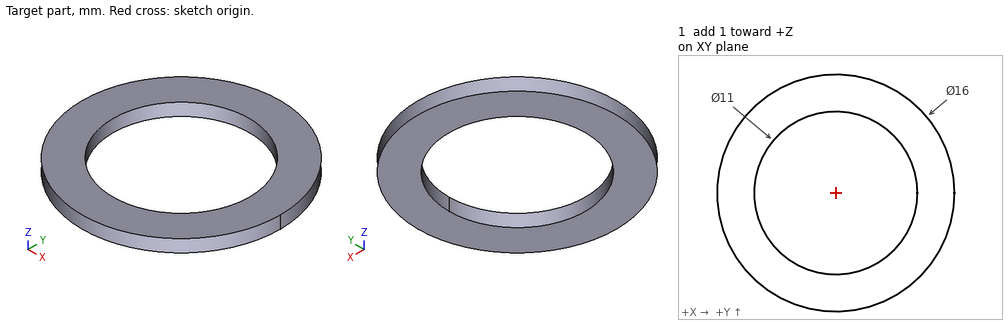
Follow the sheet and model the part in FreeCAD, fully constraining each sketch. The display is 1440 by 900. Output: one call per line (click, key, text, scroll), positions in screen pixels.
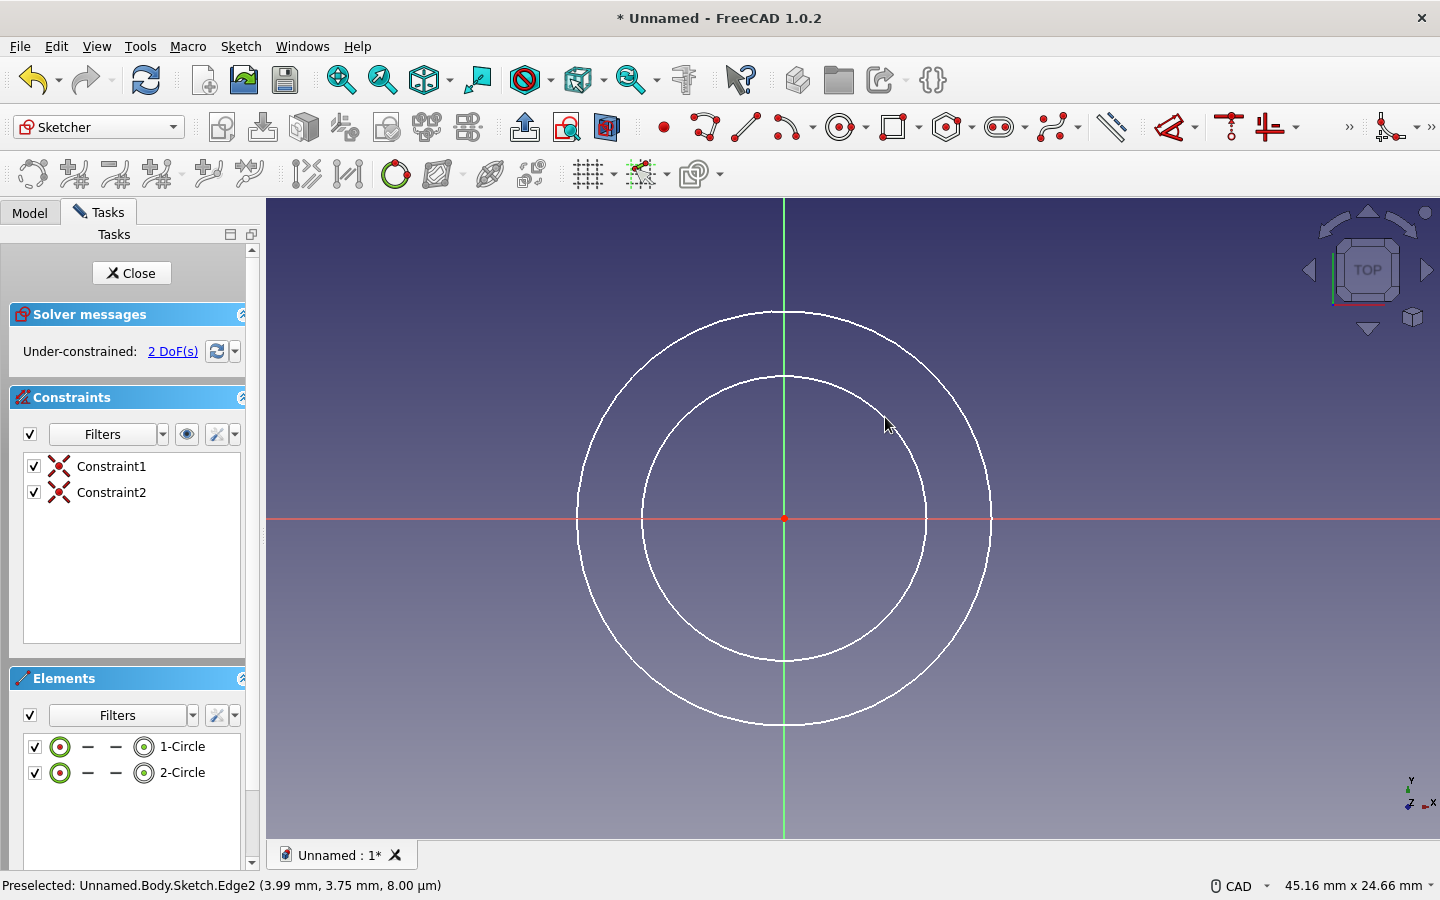
click(930, 371)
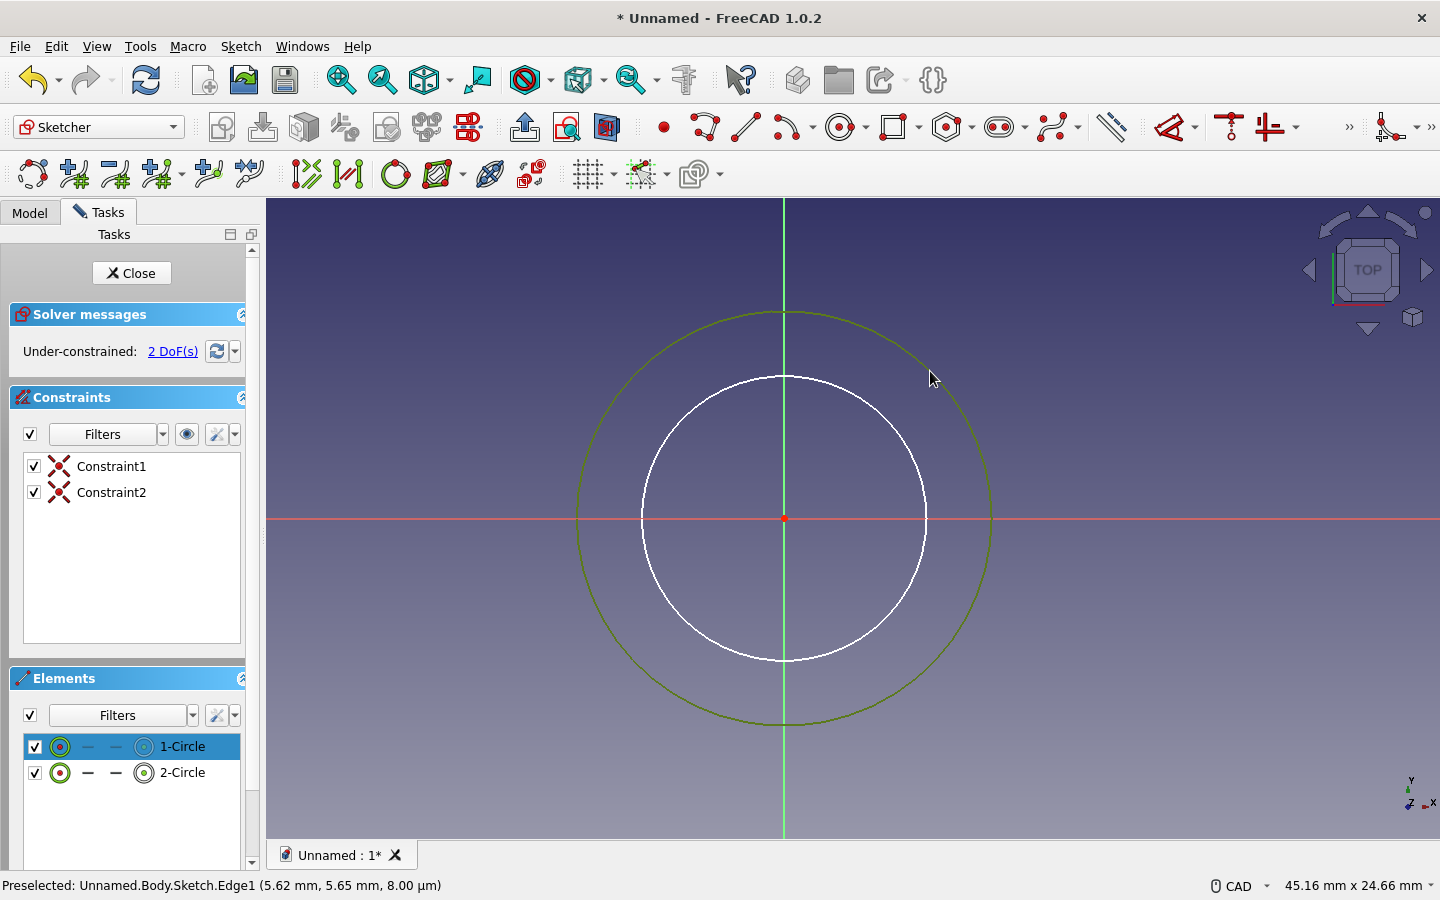
click(1194, 128)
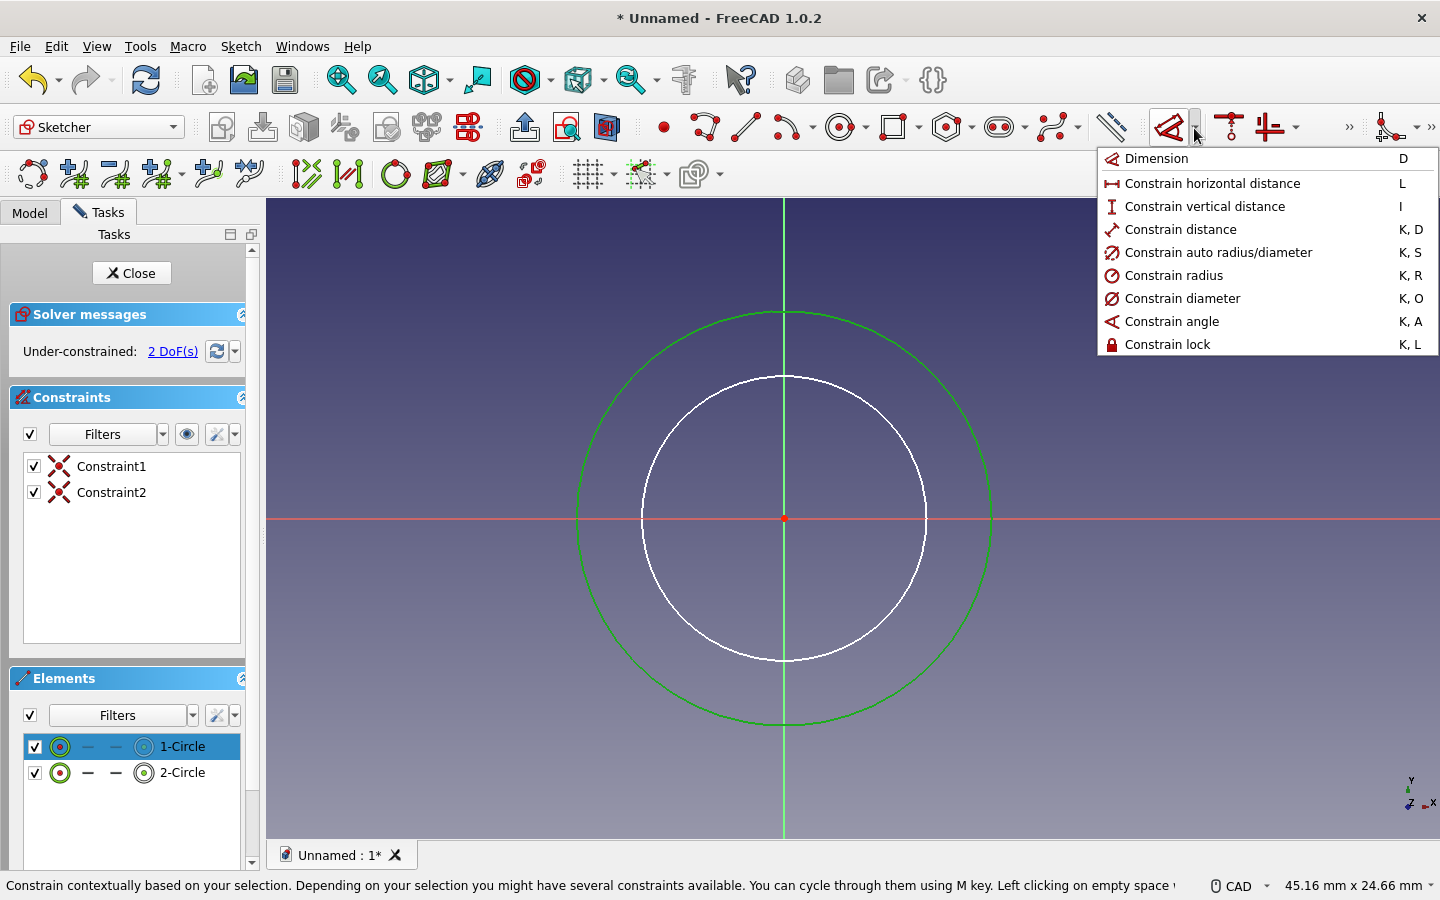
click(1268, 298)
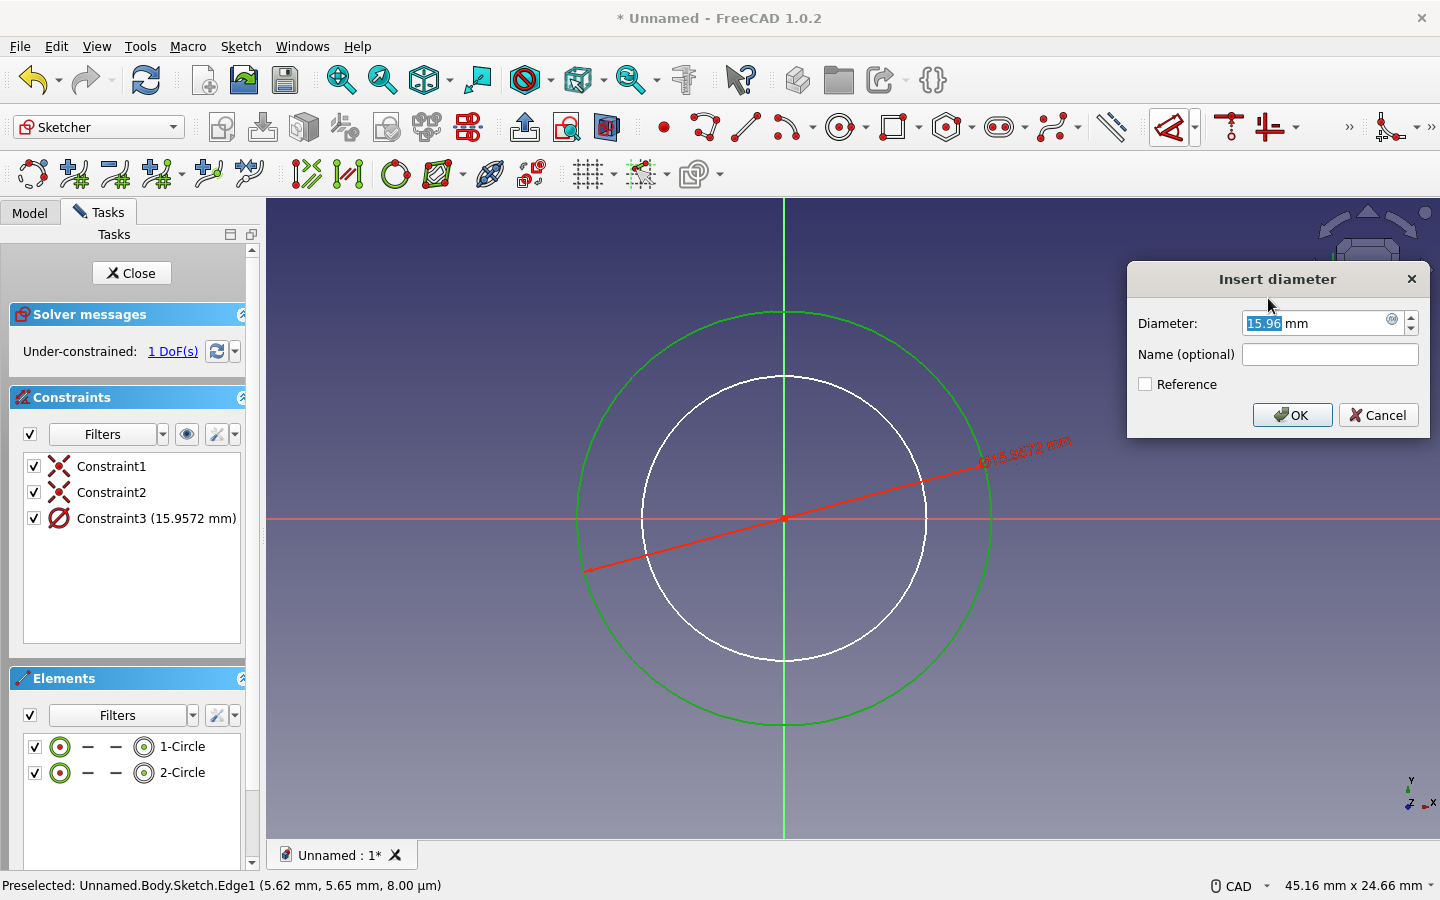
text(16)
key(Return)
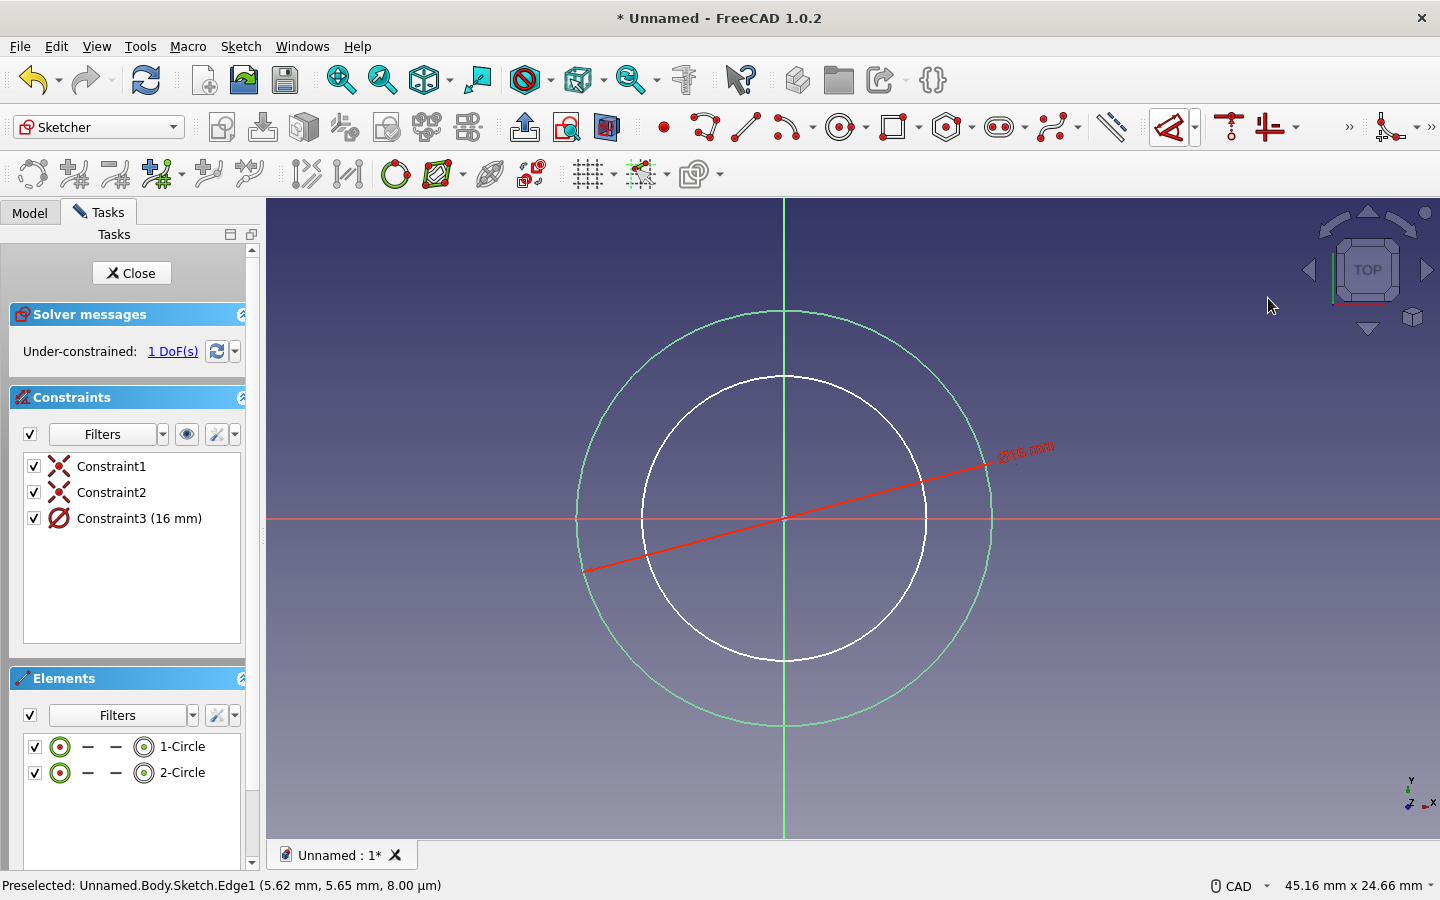
click(885, 418)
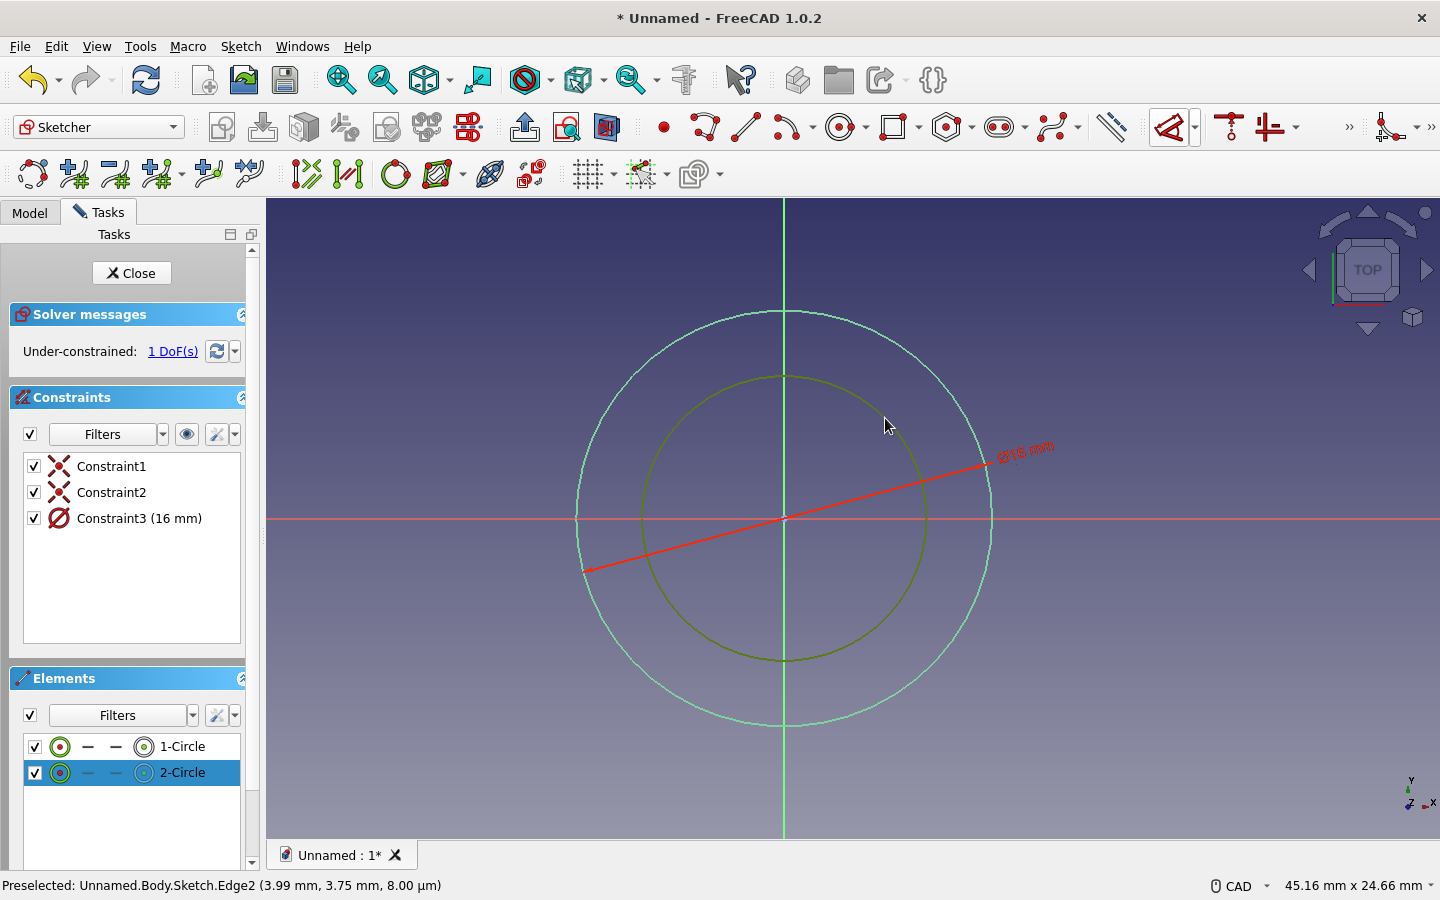
key(k)
key(o)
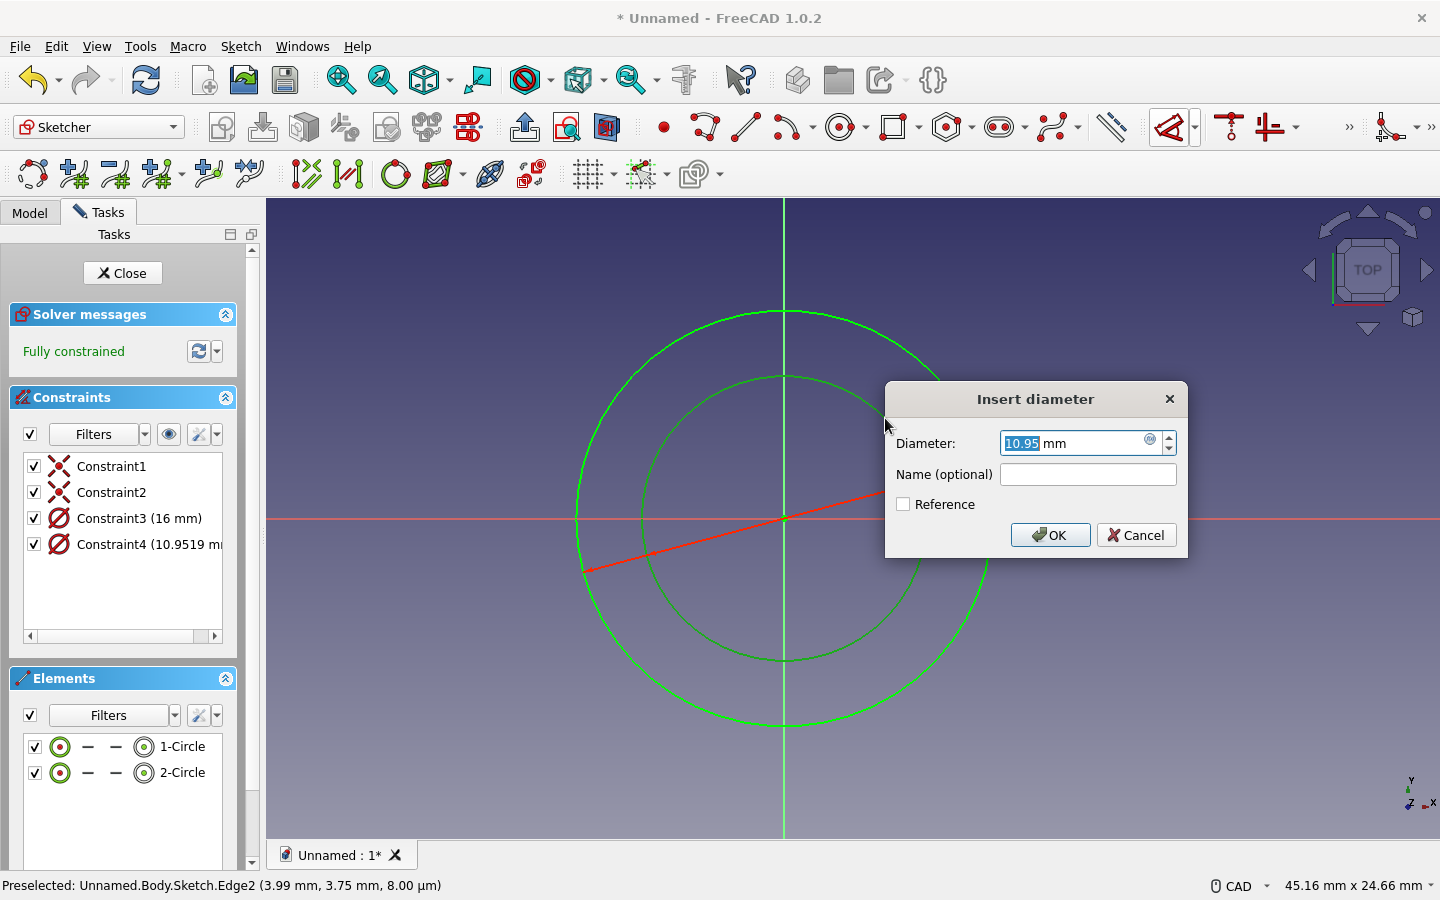
text(11)
key(Return)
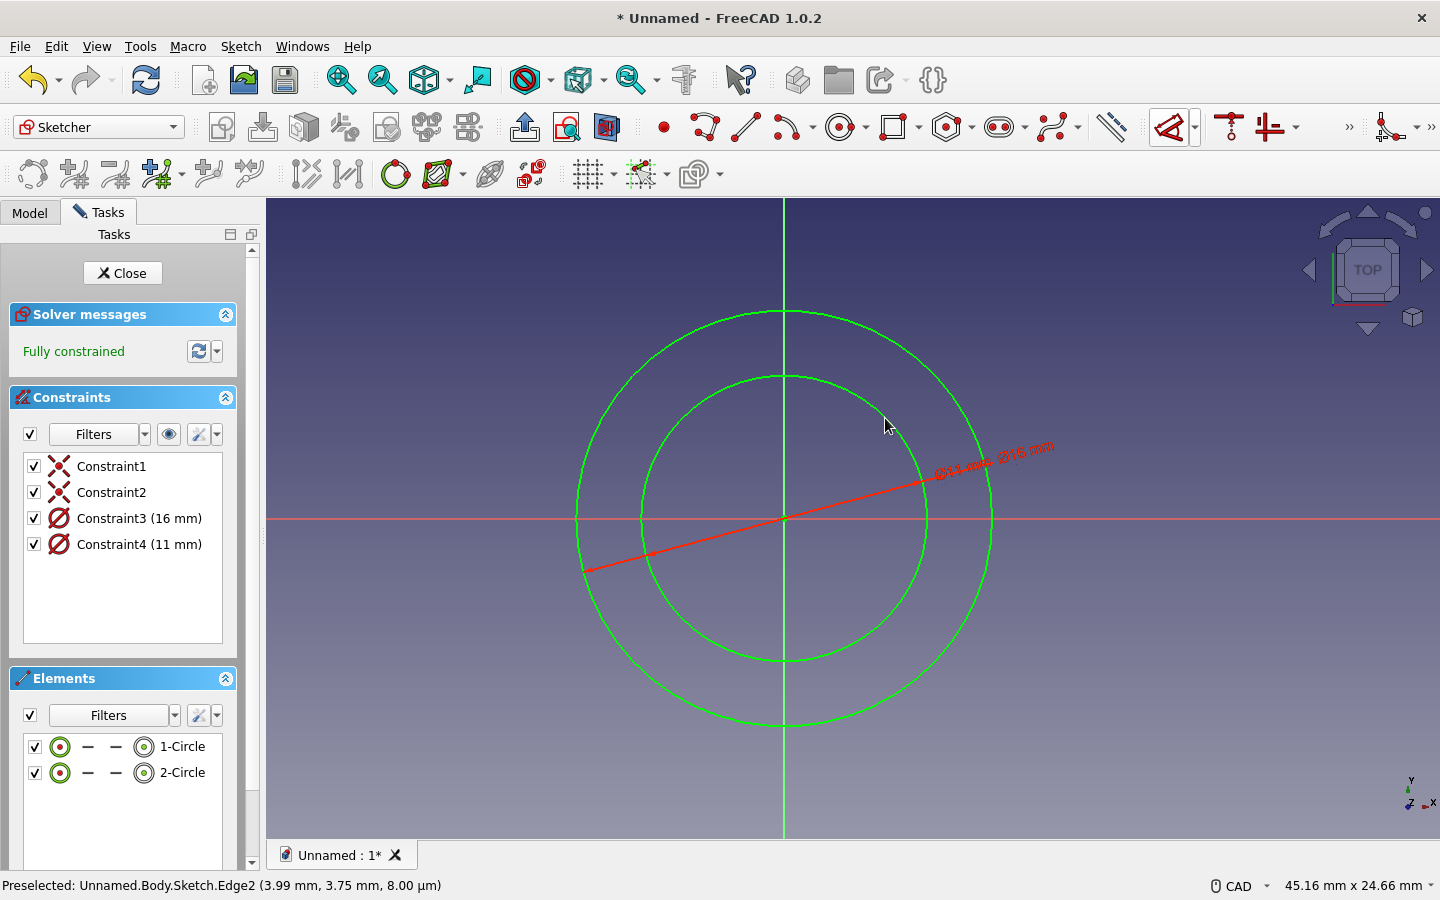
click(123, 273)